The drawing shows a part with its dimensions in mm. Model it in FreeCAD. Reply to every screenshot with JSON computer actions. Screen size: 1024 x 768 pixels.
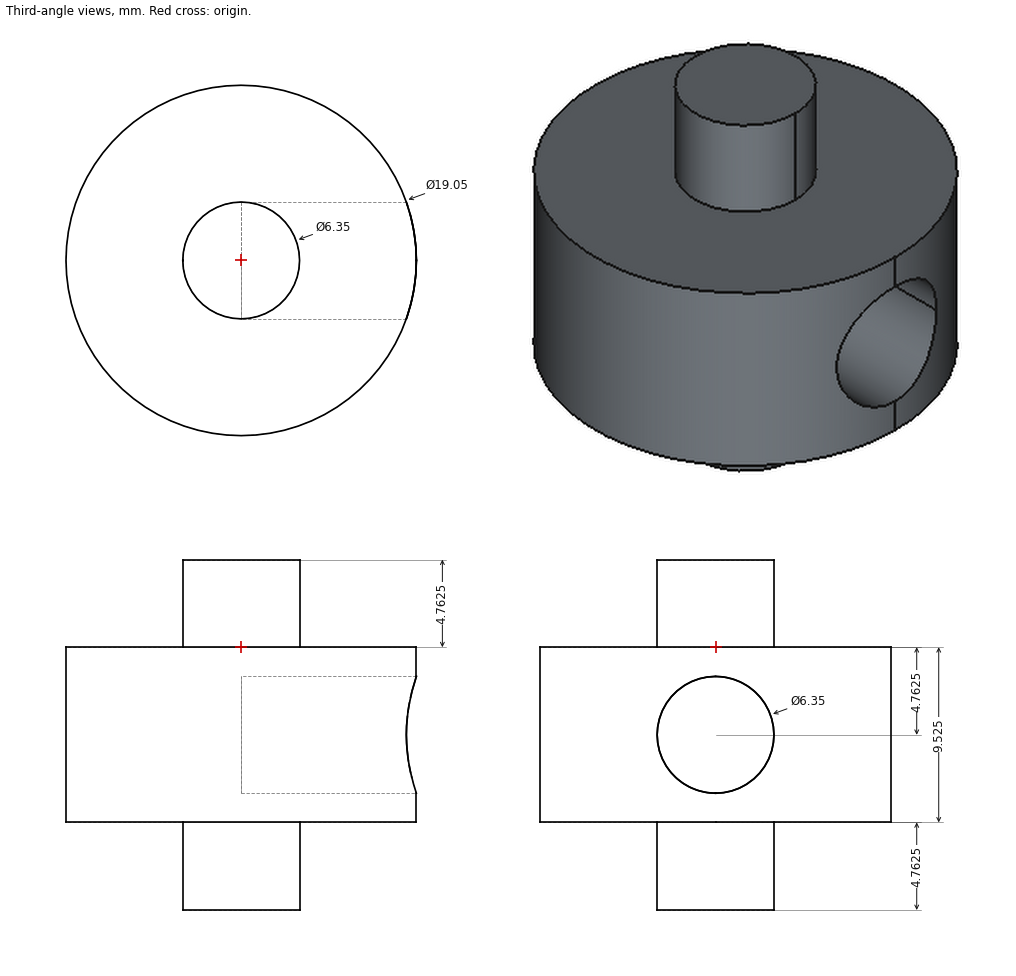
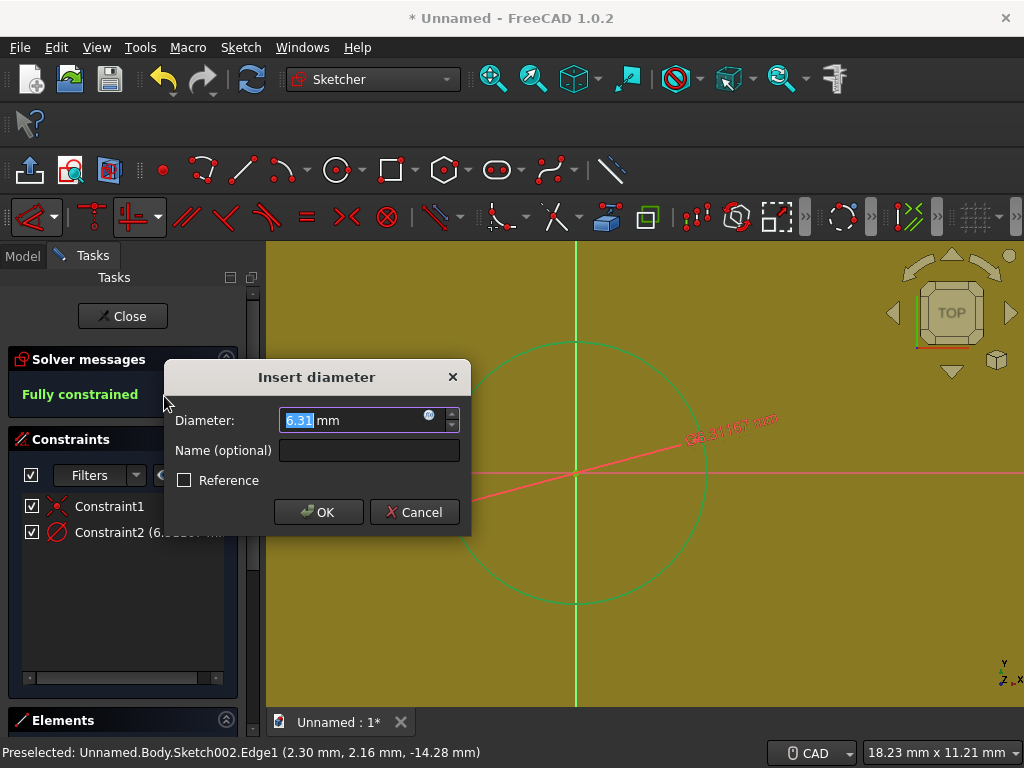
{"action": "type", "text": "6.35"}
{"action": "key", "text": "Return"}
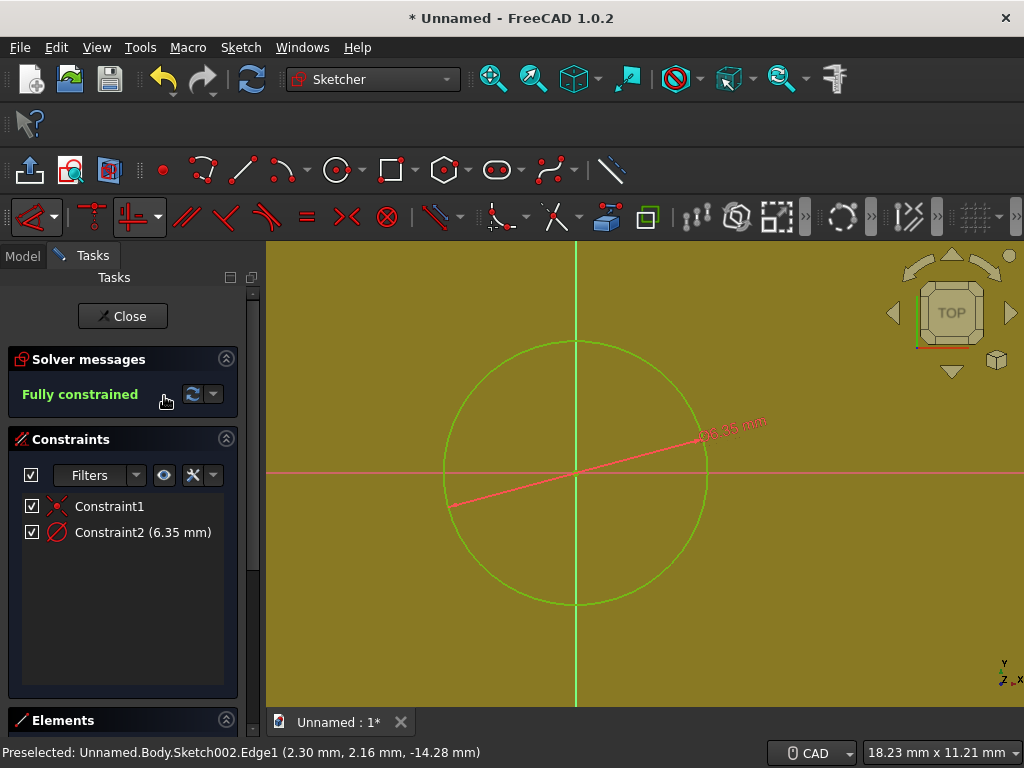
{"action": "left_click", "coordinate": [123, 316]}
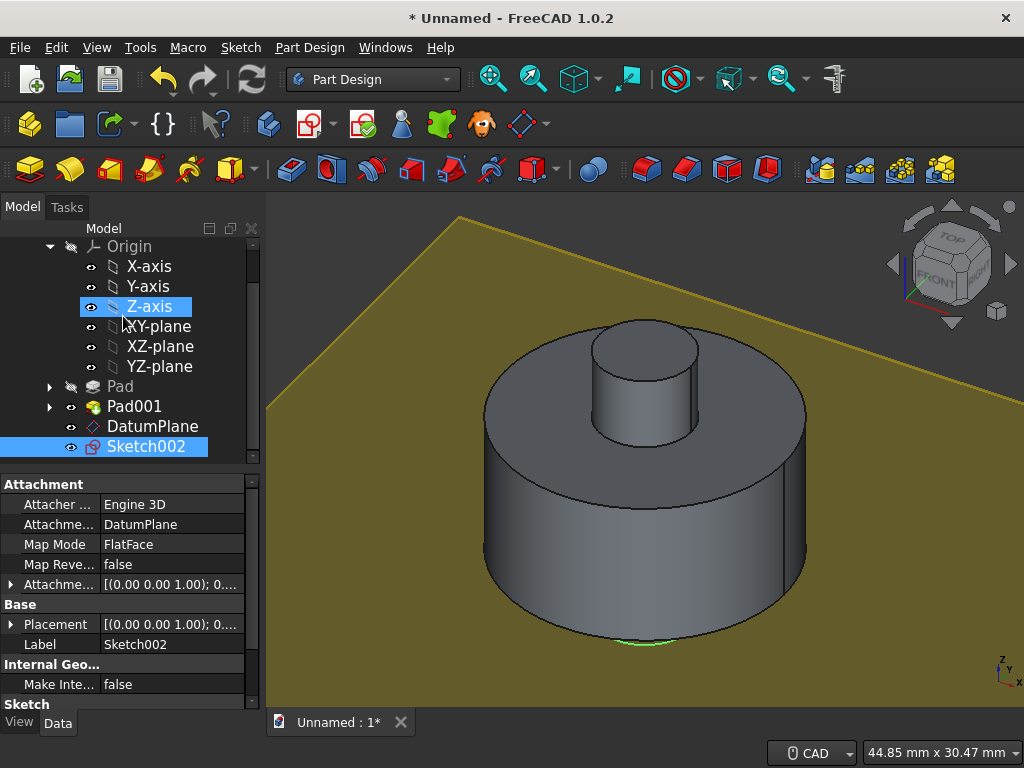
{"action": "left_click", "coordinate": [30, 170]}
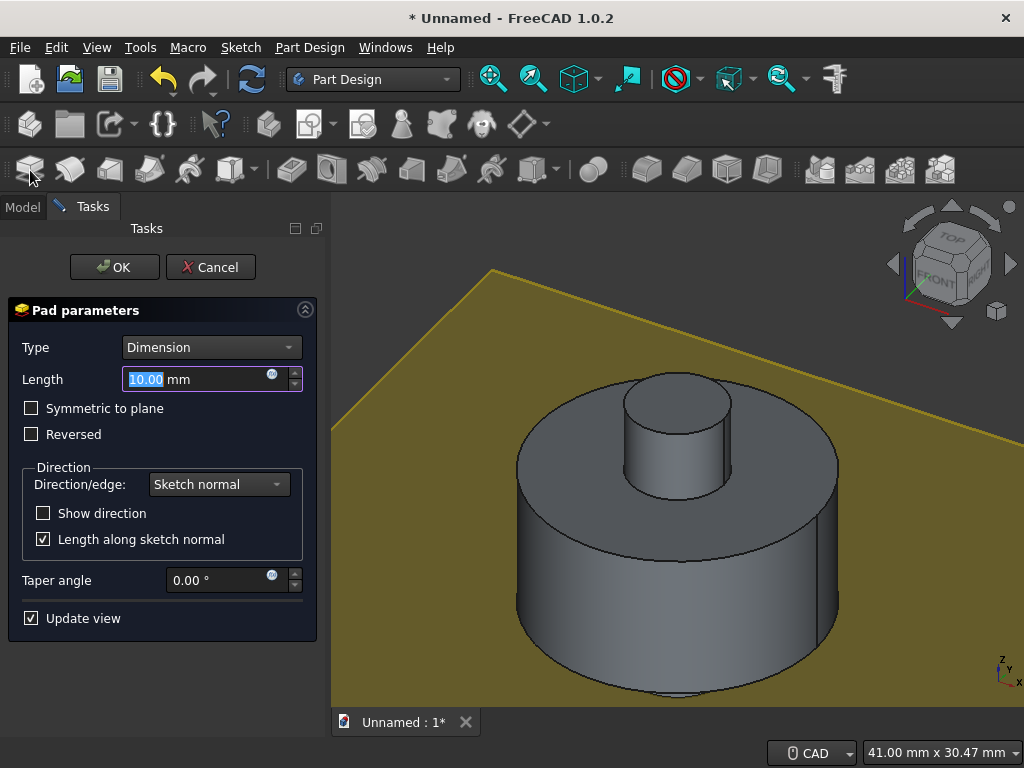
{"action": "type", "text": "4.7625"}
{"action": "key", "text": "Tab"}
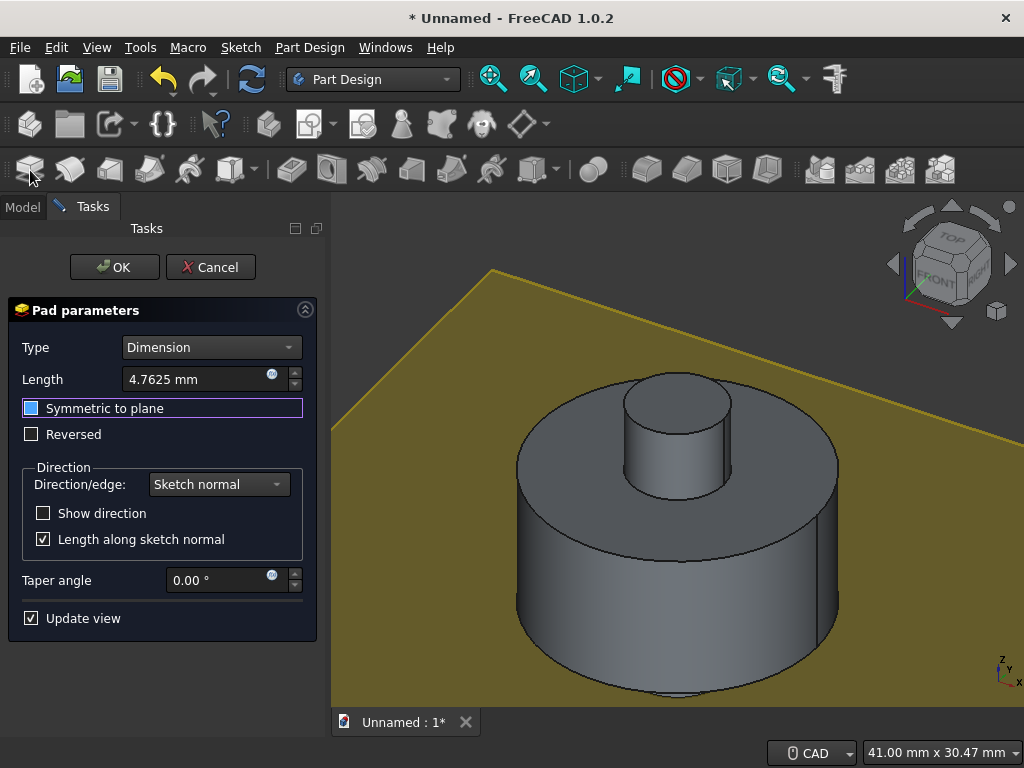
{"action": "left_click", "coordinate": [115, 267]}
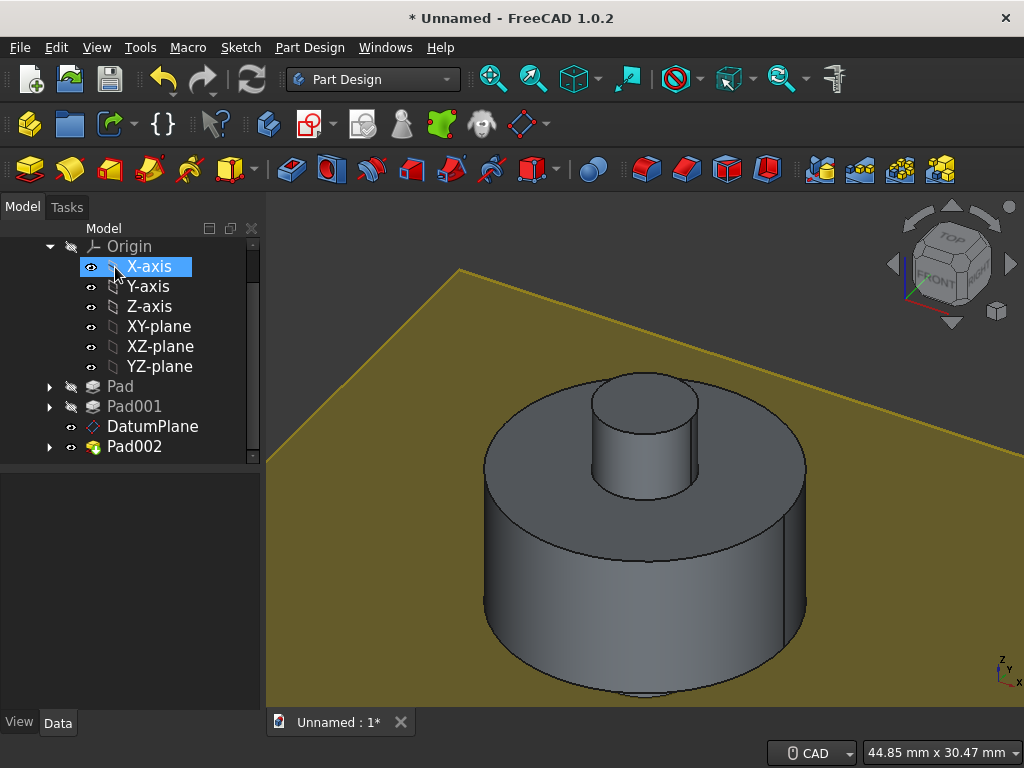
{"action": "left_click", "coordinate": [116, 427]}
{"action": "key", "text": "space"}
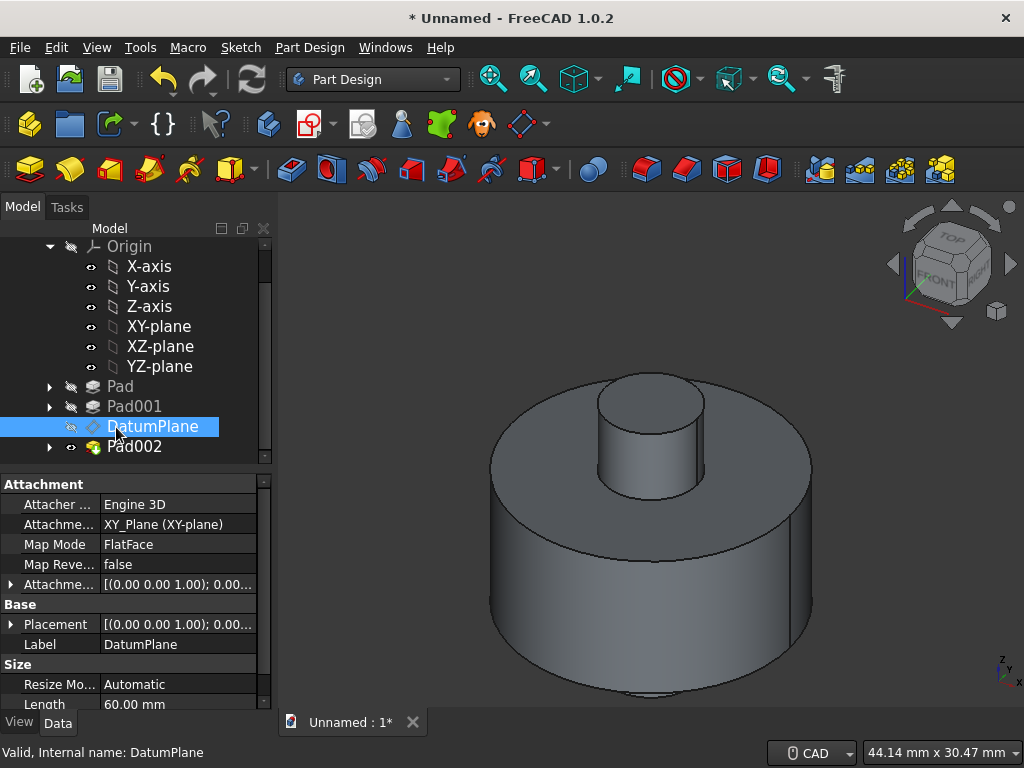
{"action": "key", "text": "v f"}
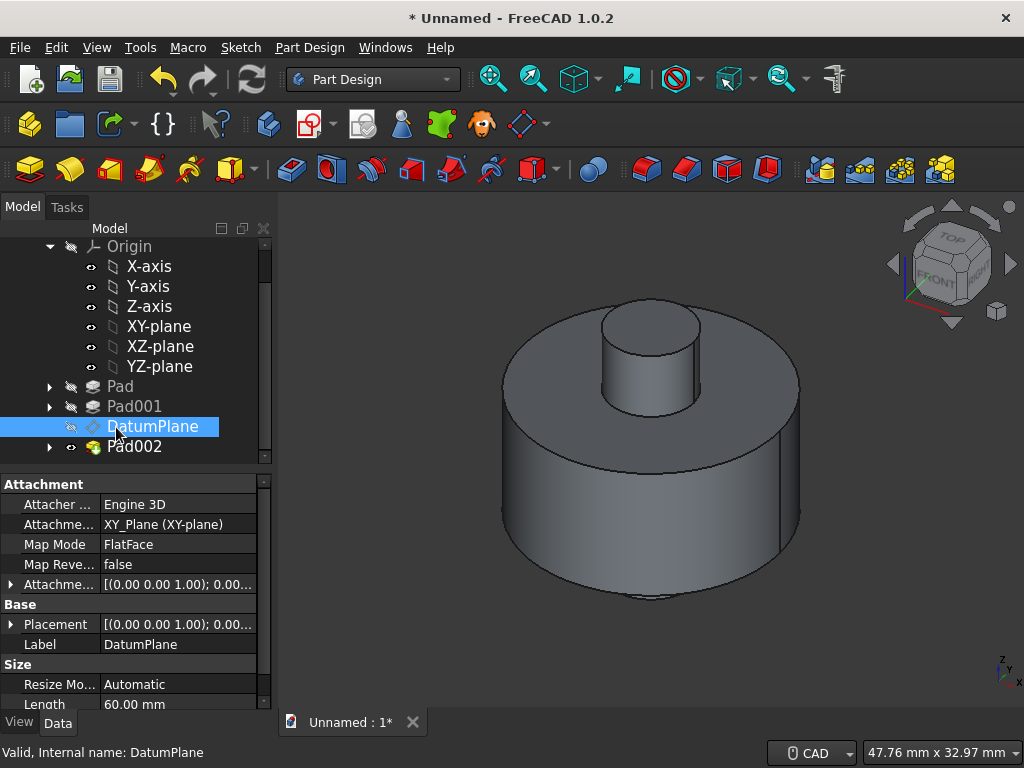
{"action": "left_click", "coordinate": [318, 667]}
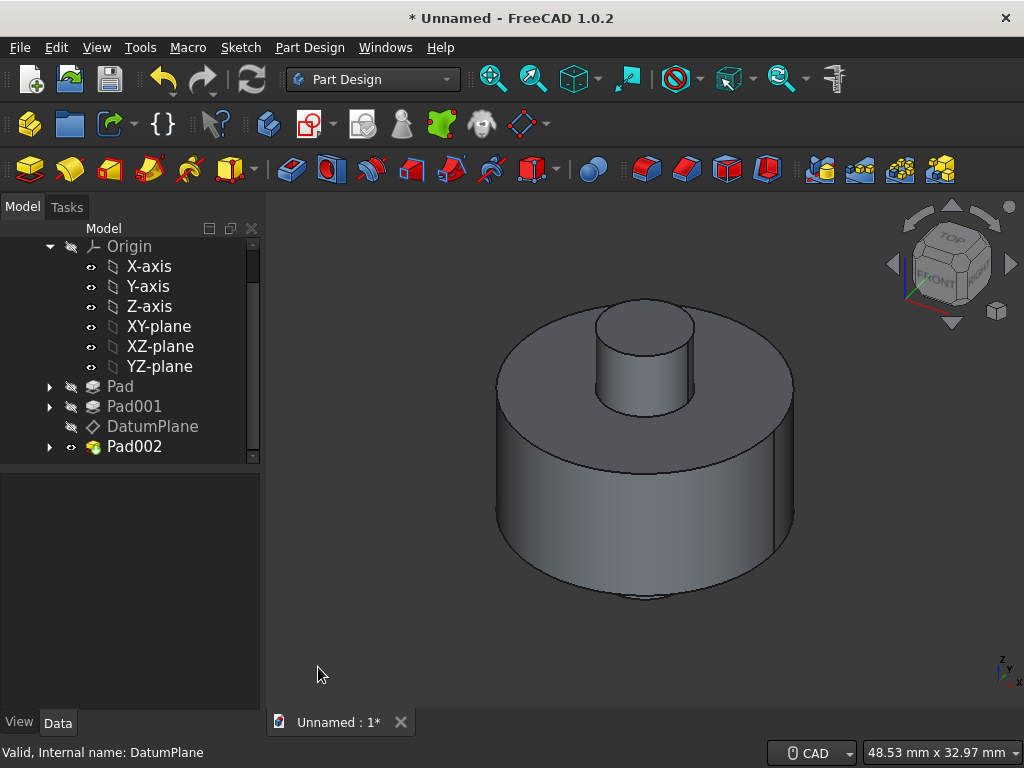
{"action": "left_click", "coordinate": [310, 124]}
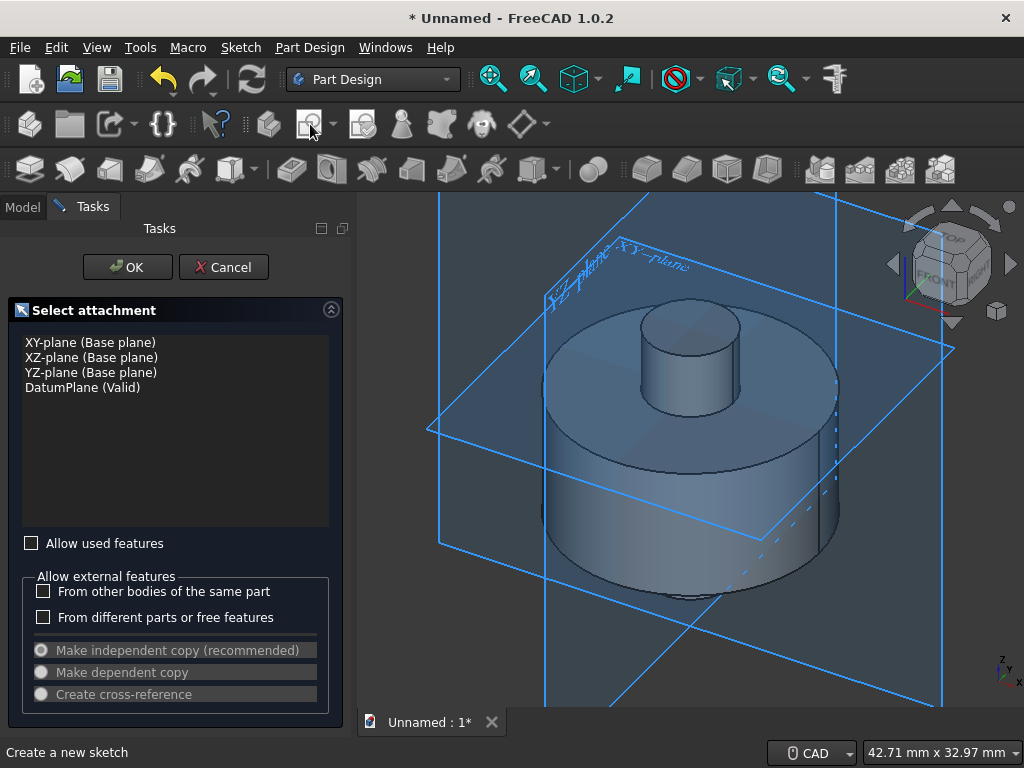
{"action": "left_click", "coordinate": [82, 372]}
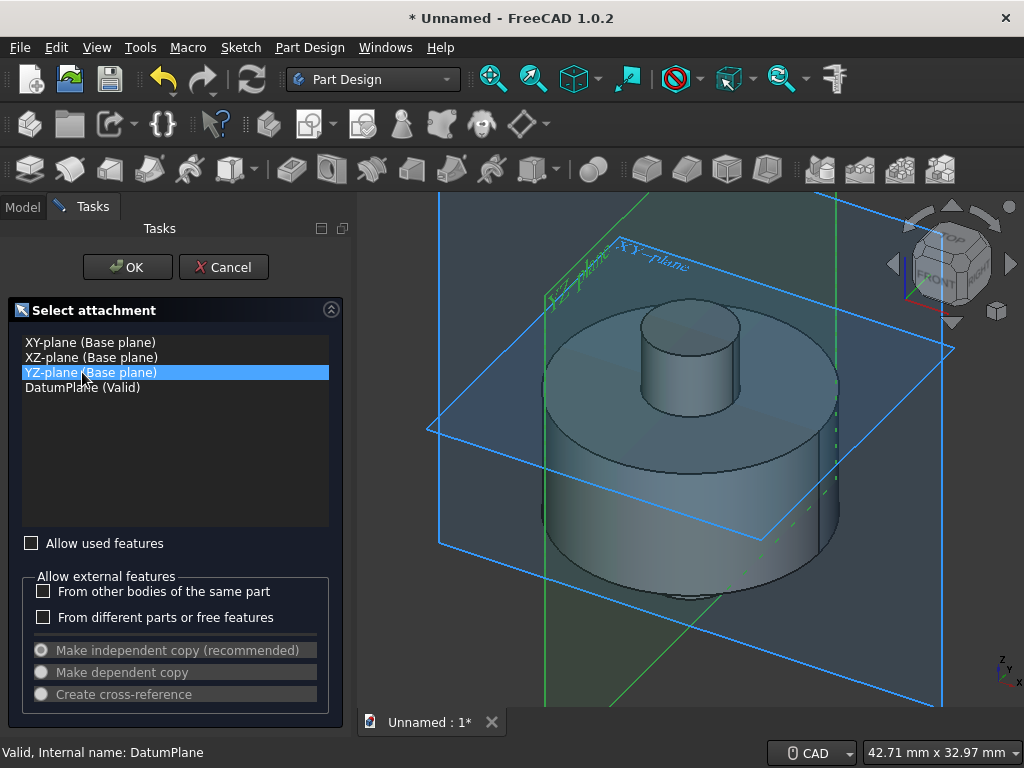
{"action": "left_click", "coordinate": [128, 267]}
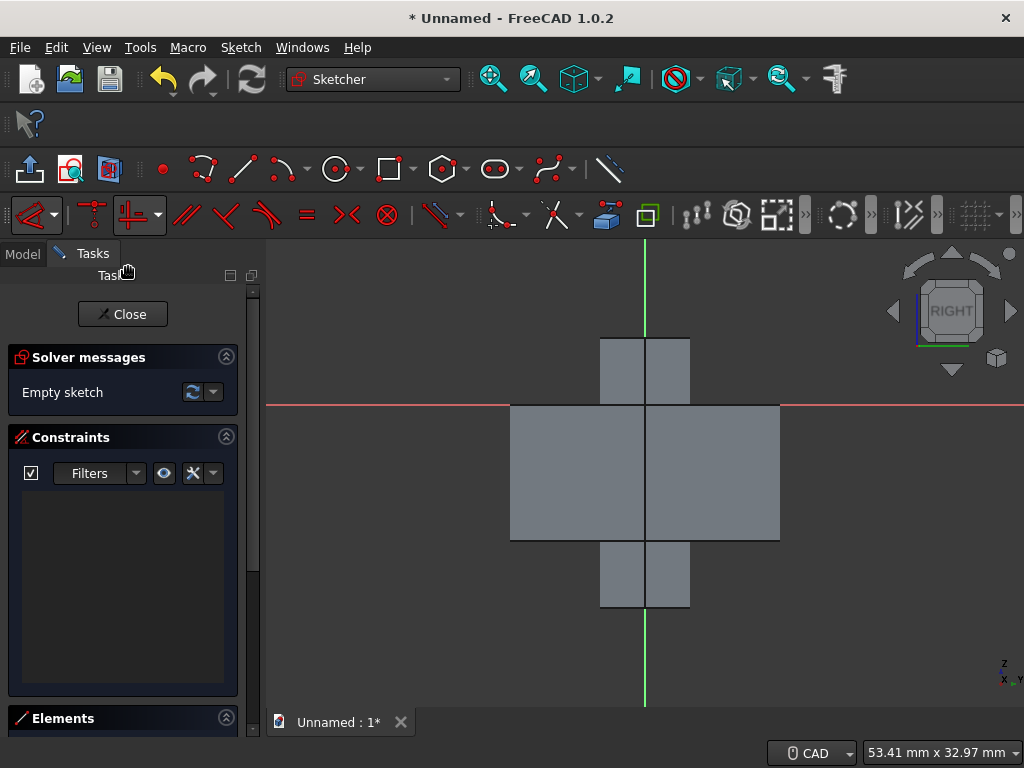
{"action": "key", "text": "q s"}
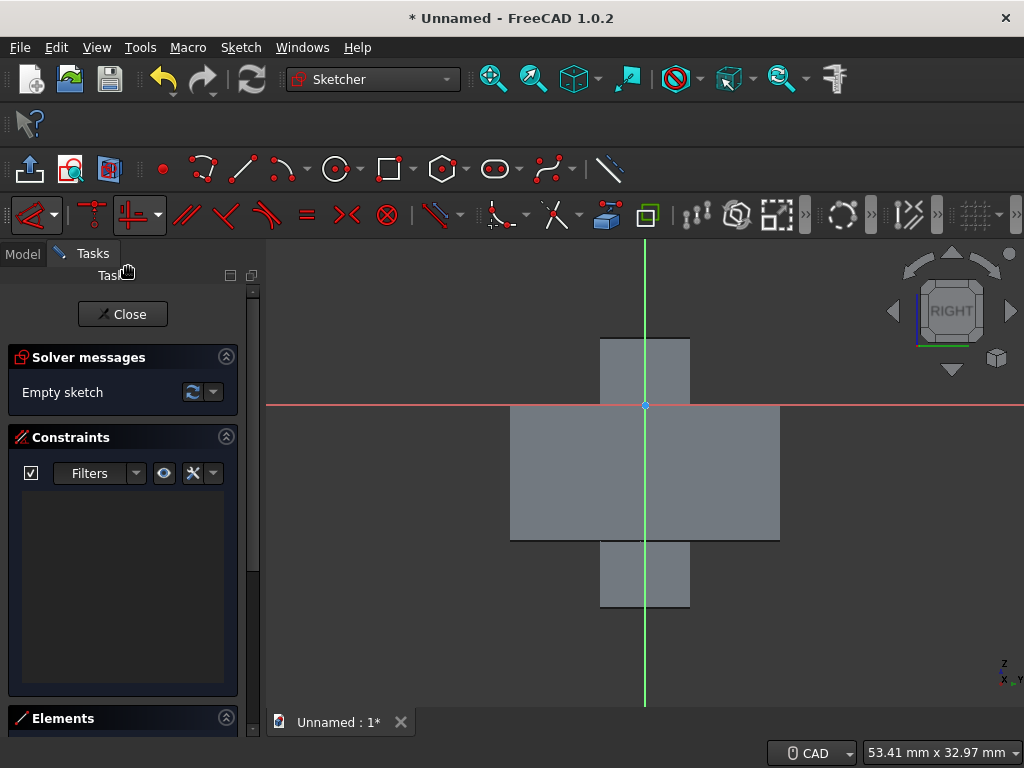
{"action": "scroll", "coordinate": [685, 455], "scroll_direction": "up", "scroll_amount": 5}